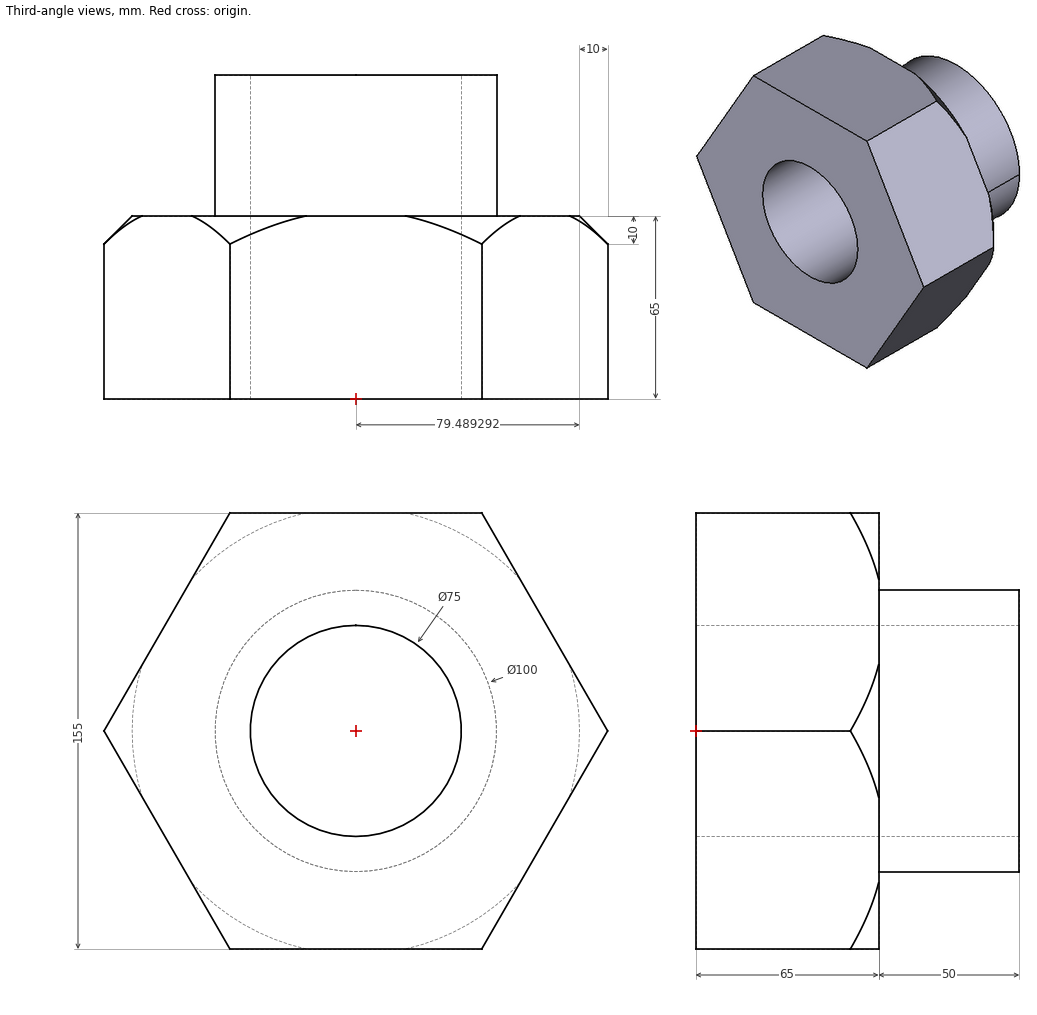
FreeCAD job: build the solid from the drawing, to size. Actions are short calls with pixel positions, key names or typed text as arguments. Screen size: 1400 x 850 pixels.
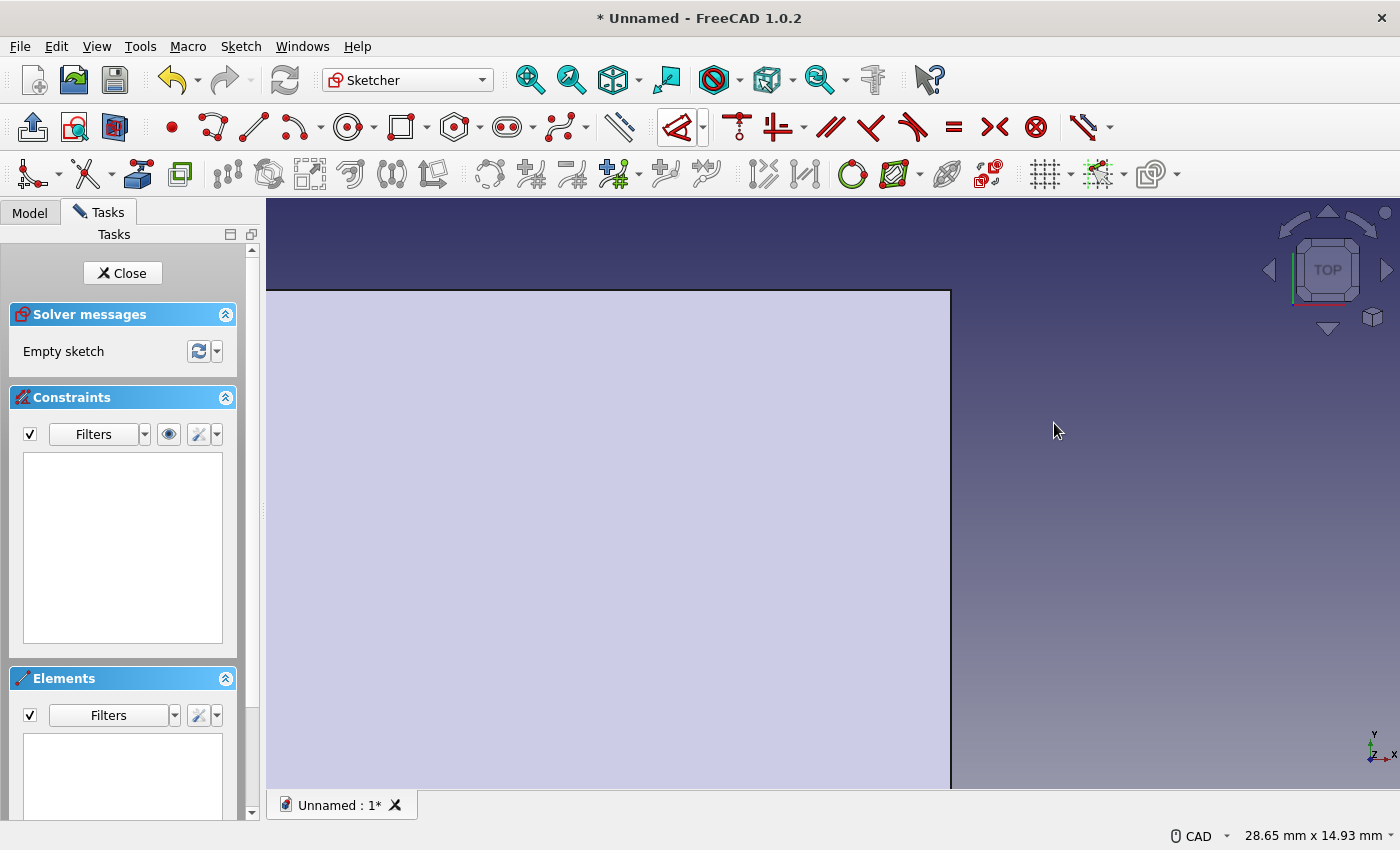
click(213, 128)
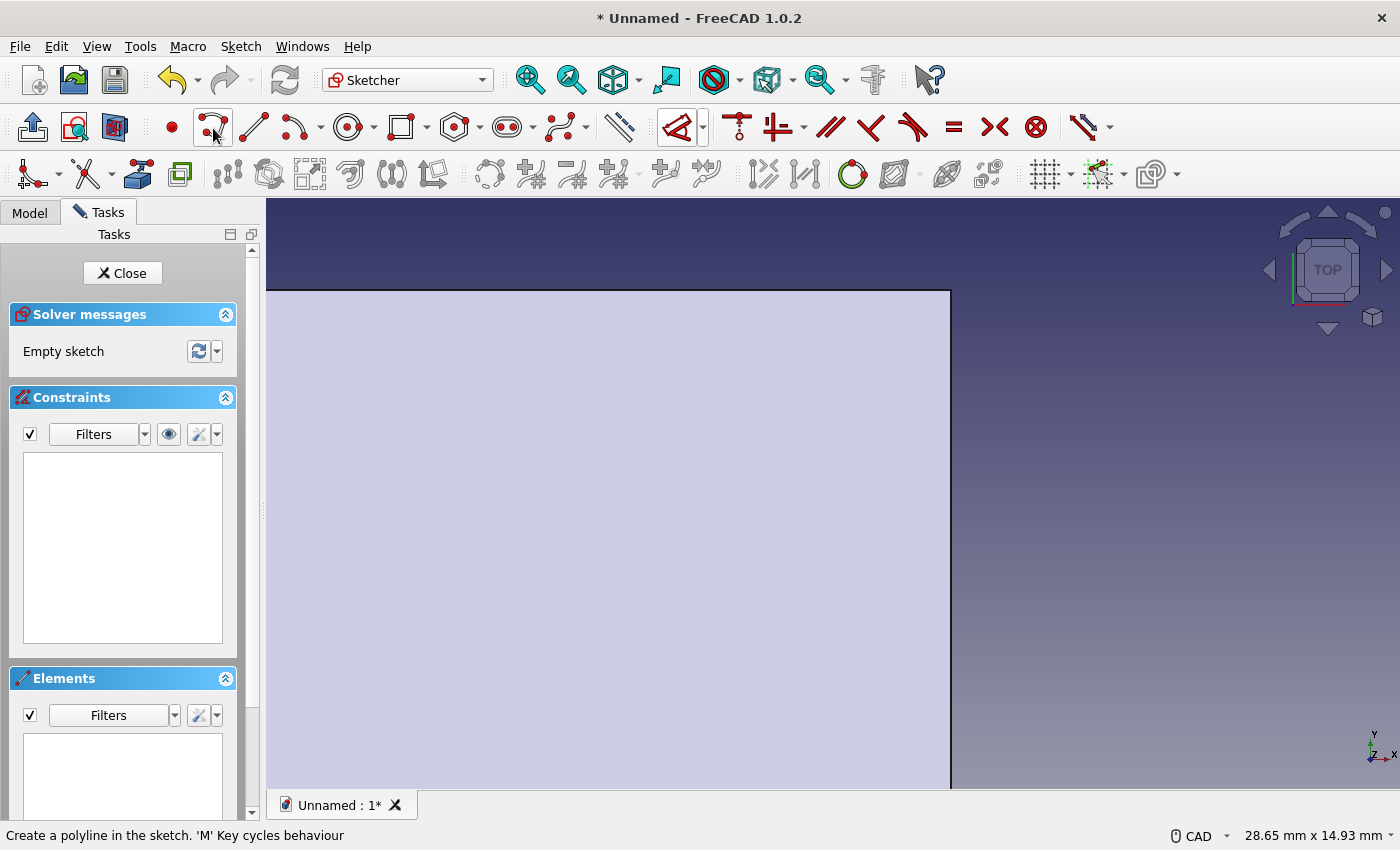
click(555, 290)
click(951, 686)
click(951, 290)
click(555, 291)
key(Escape)
key(Escape)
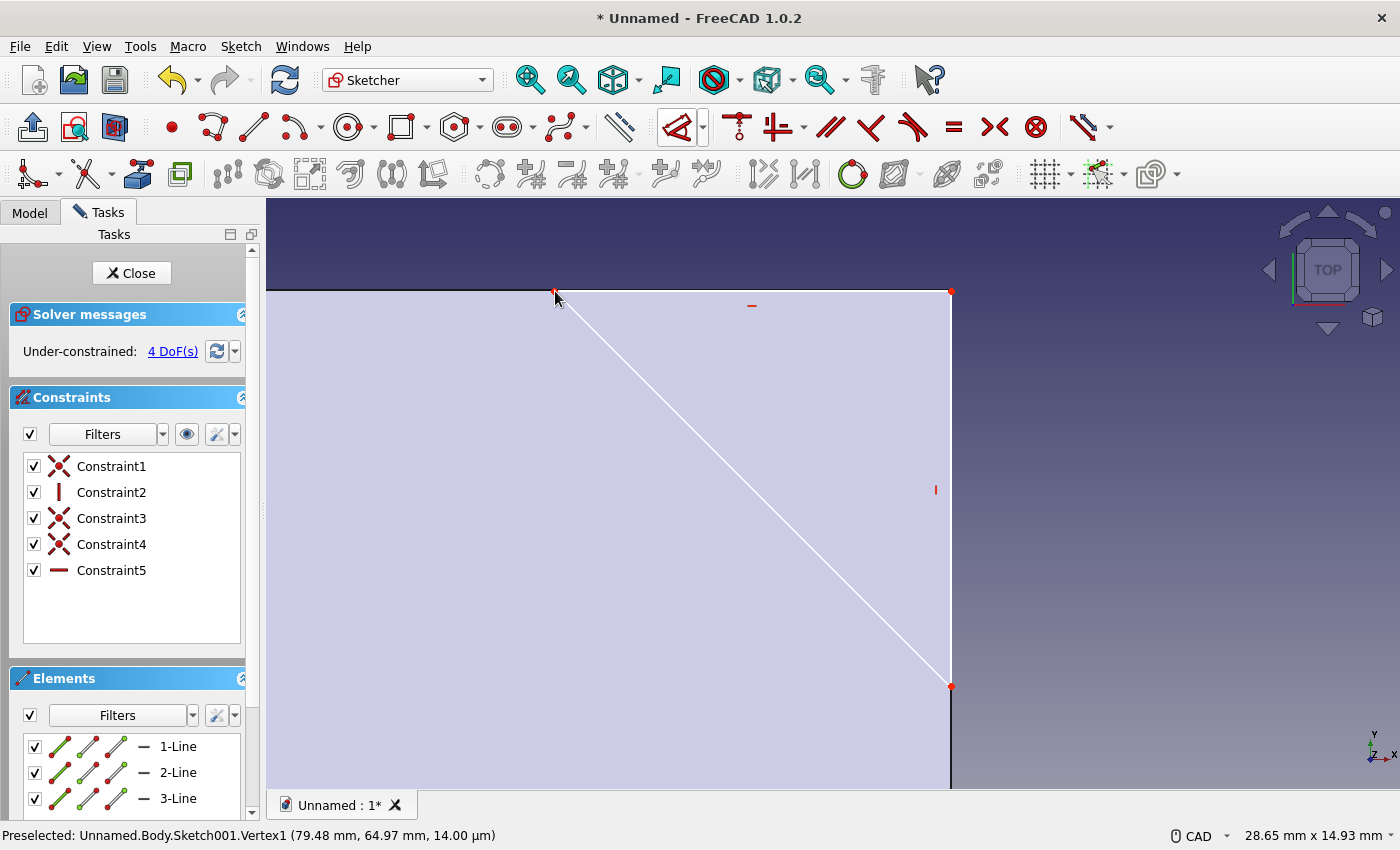
click(951, 568)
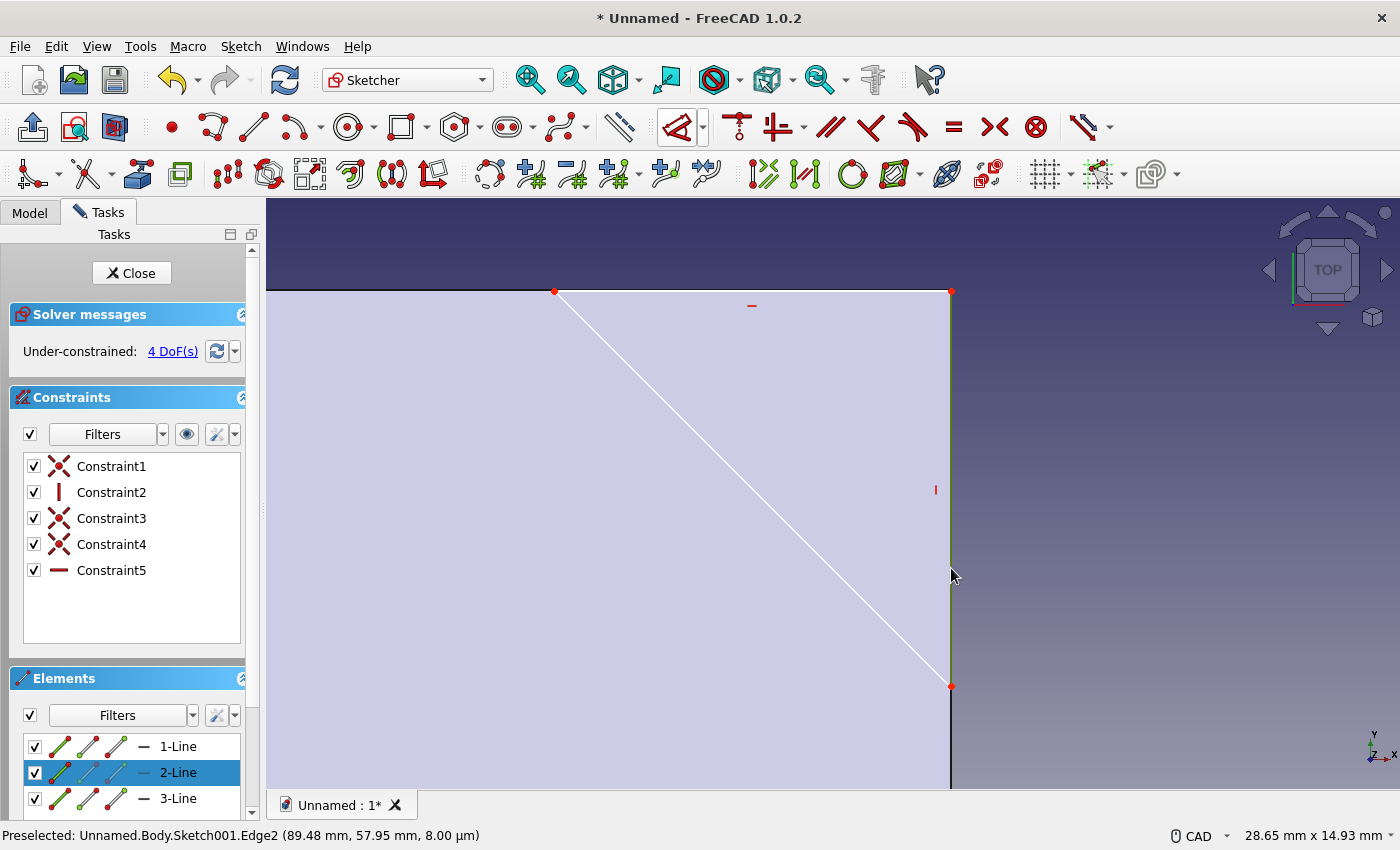
click(702, 128)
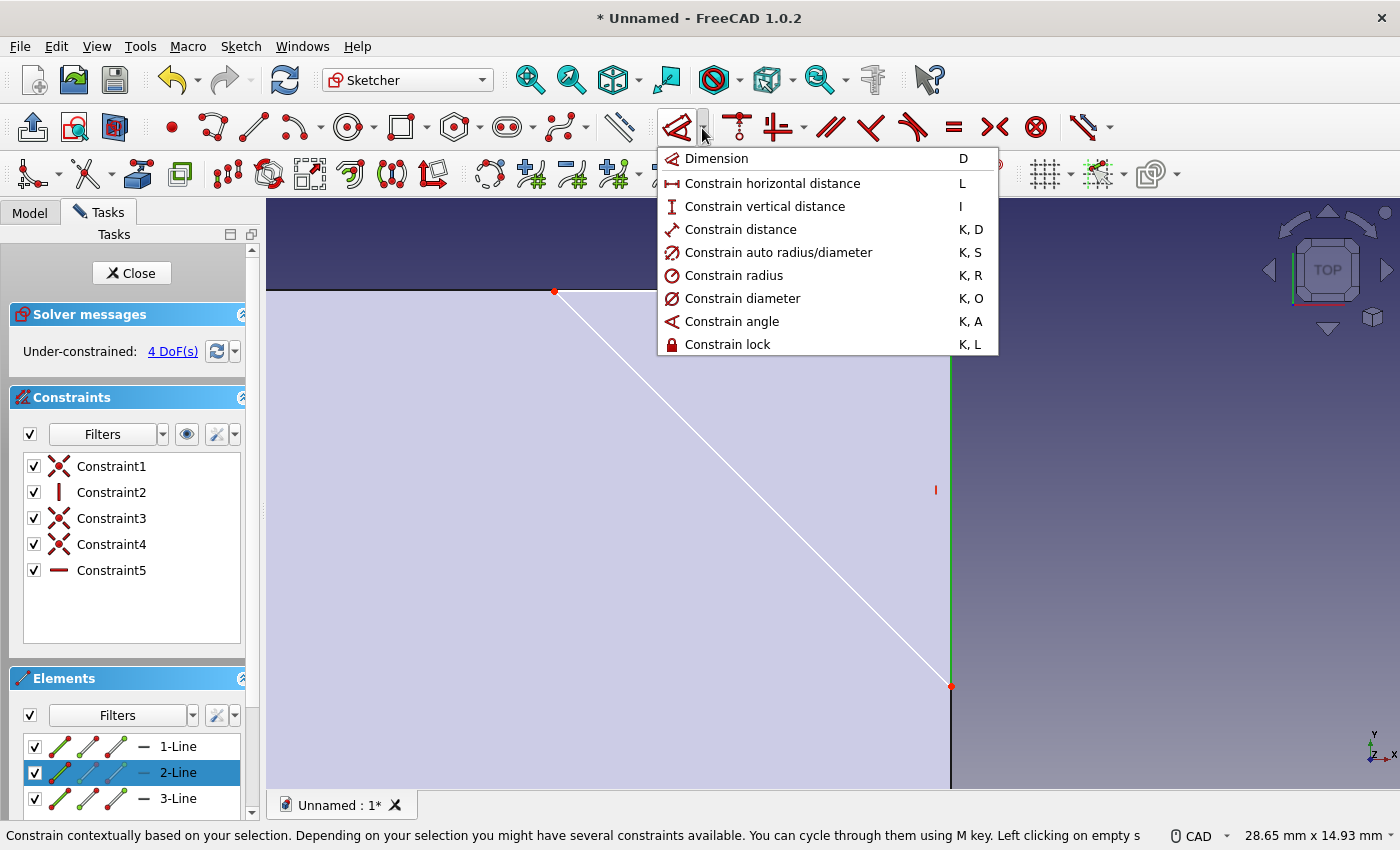
click(828, 206)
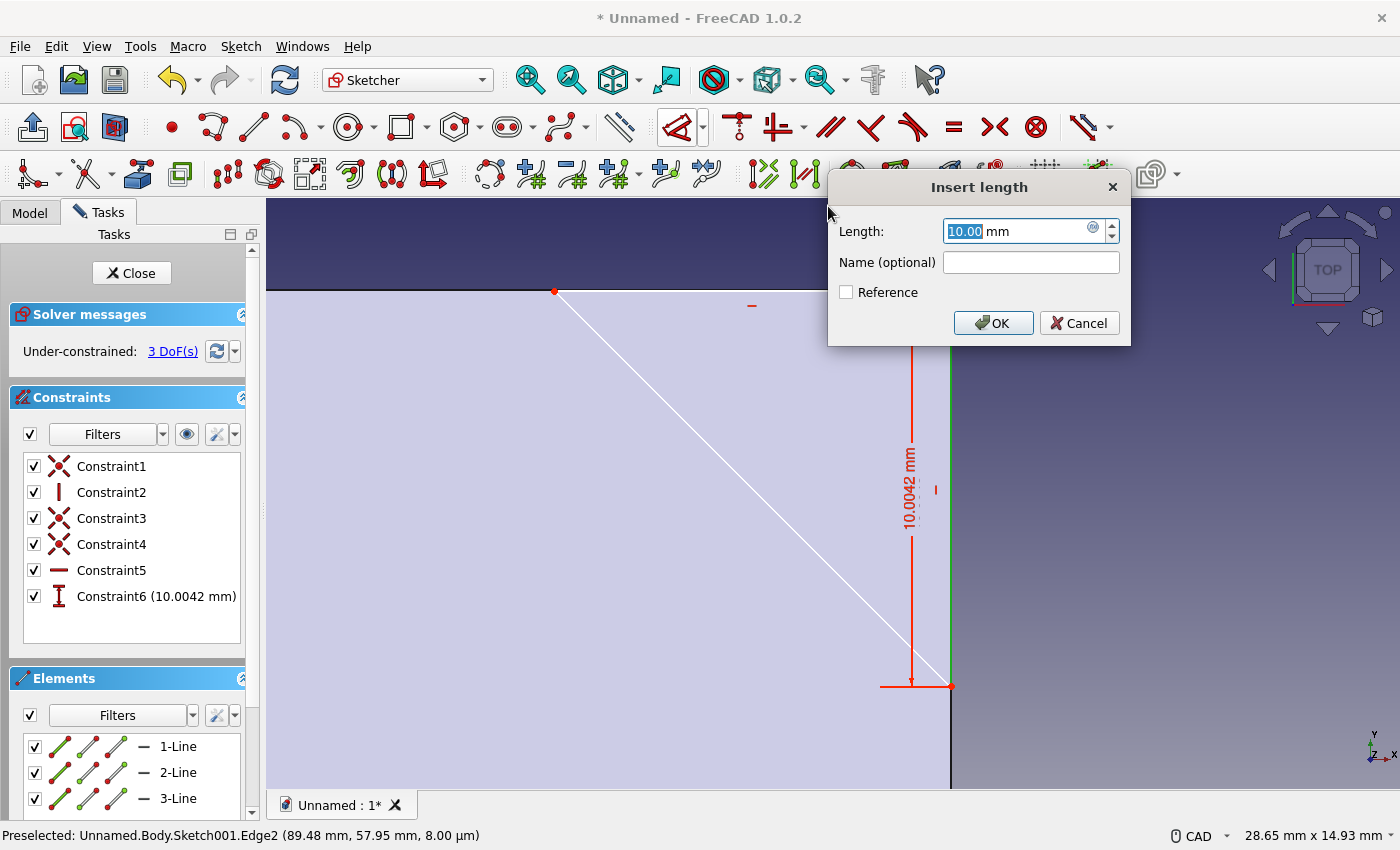
text(10)
key(Return)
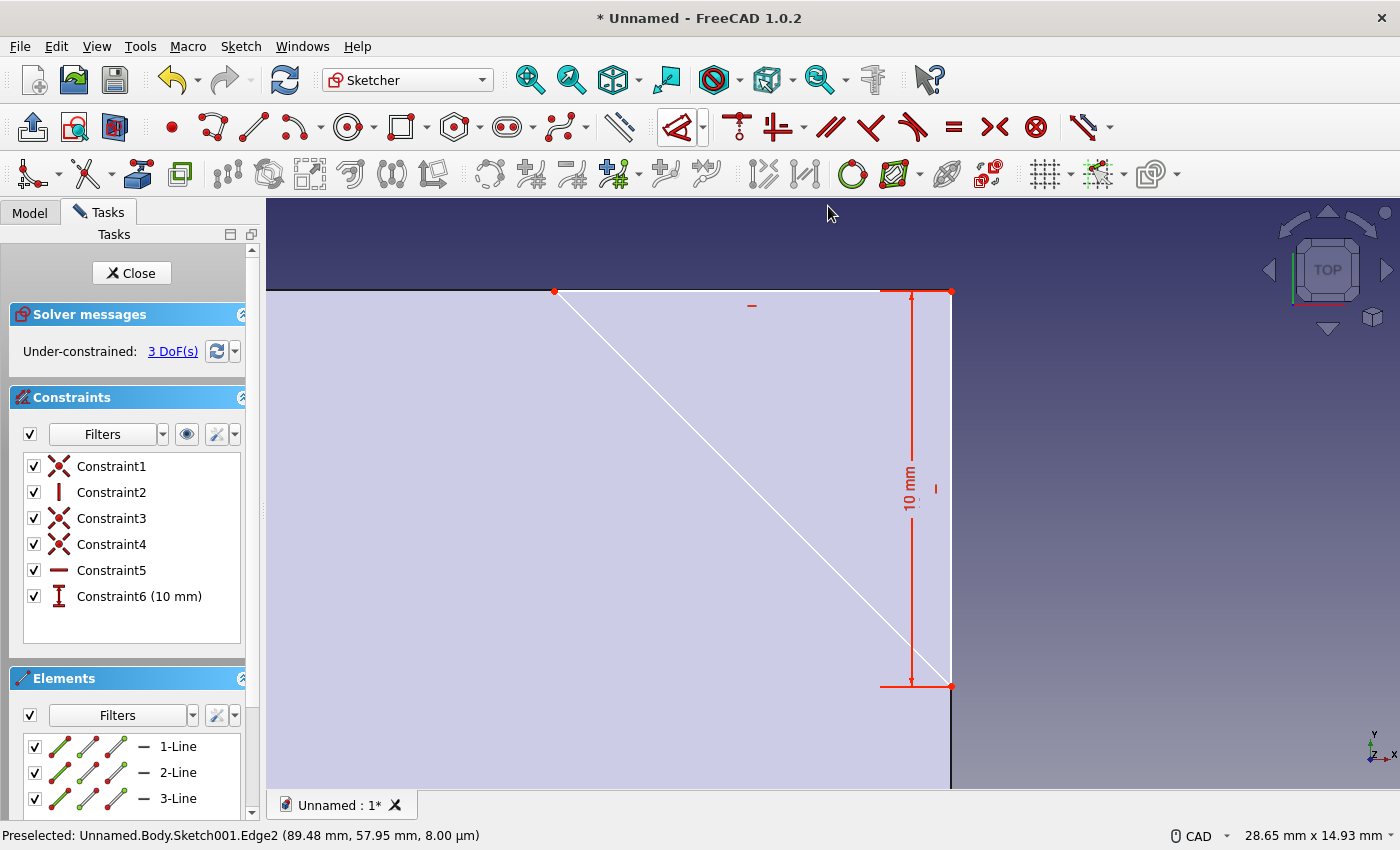
click(832, 291)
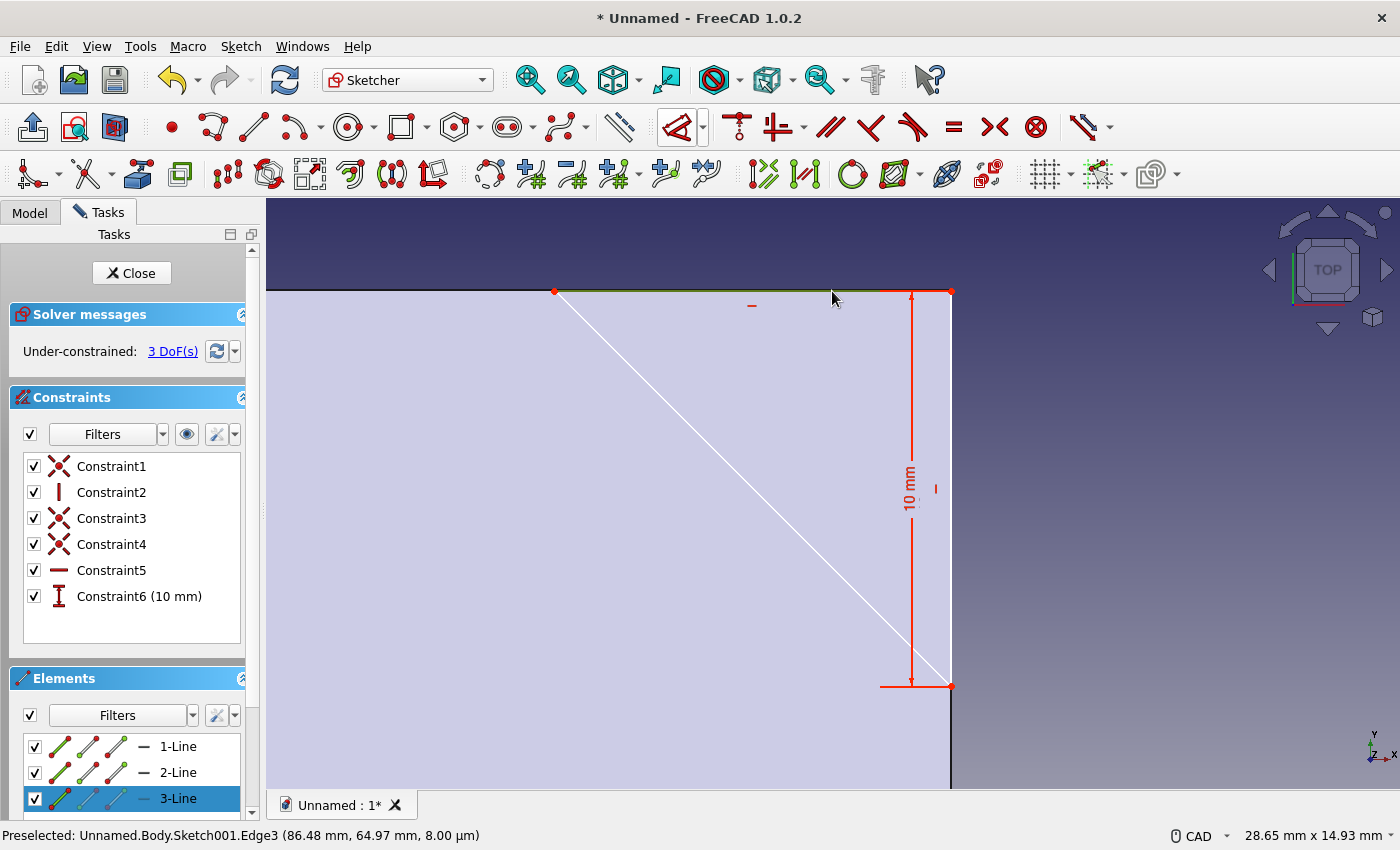
key(l)